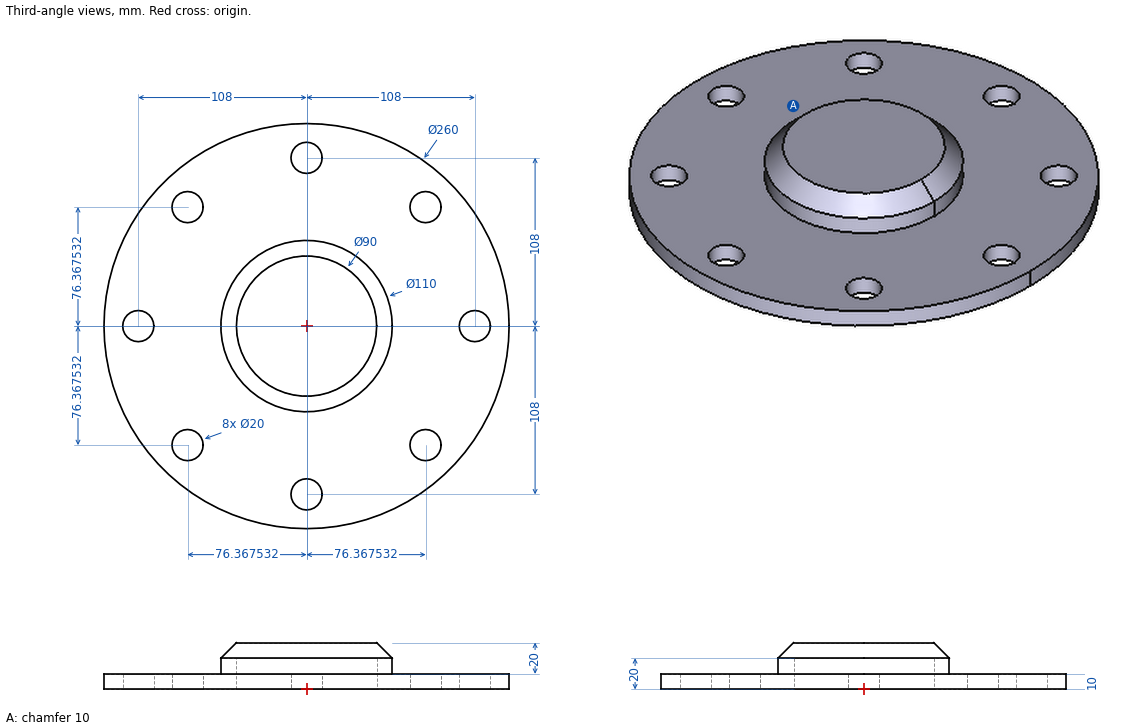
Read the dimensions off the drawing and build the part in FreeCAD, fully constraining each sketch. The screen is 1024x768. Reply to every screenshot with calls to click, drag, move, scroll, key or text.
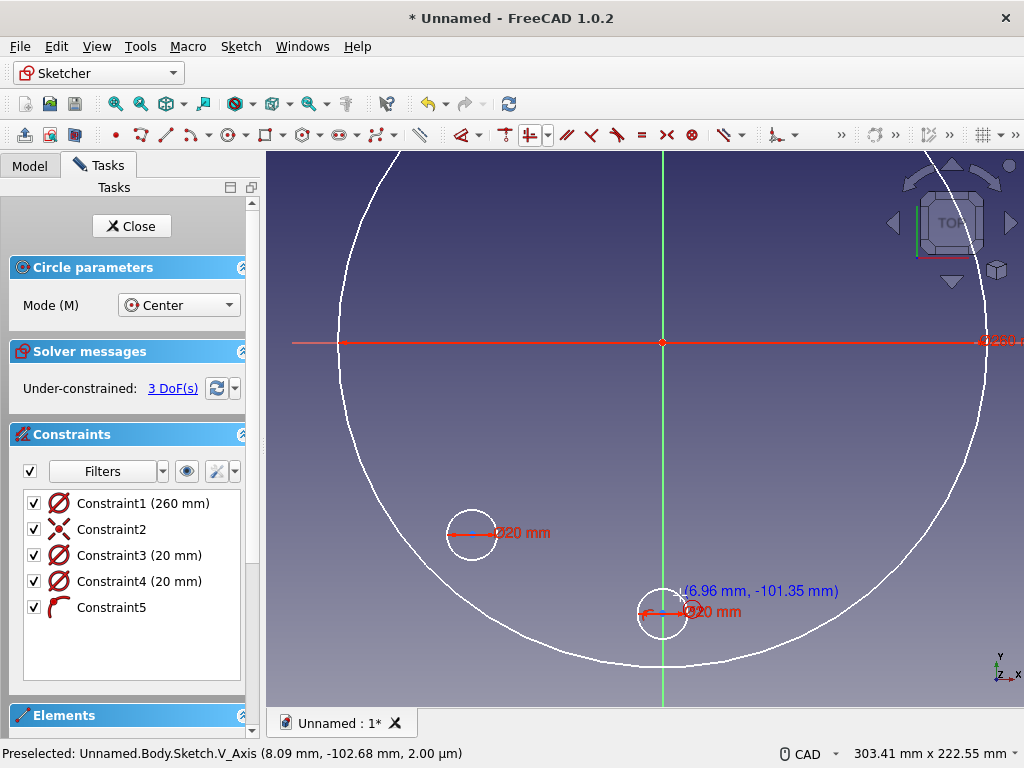
click(853, 534)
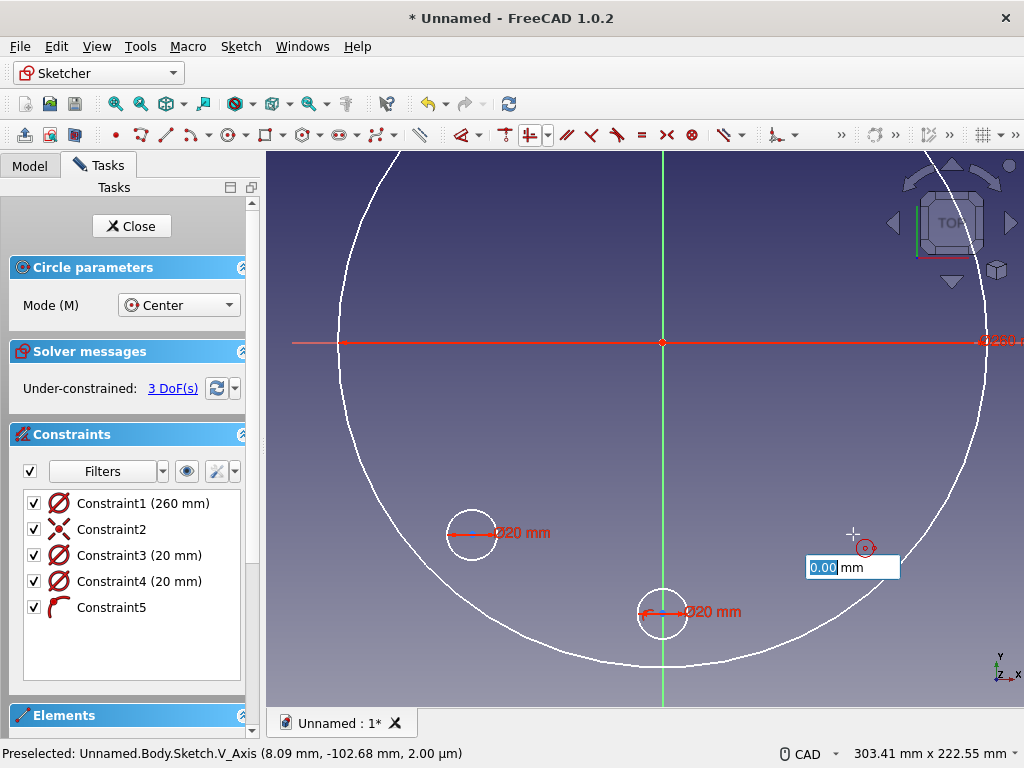
scroll(472, 534, down, 3)
move(691, 524)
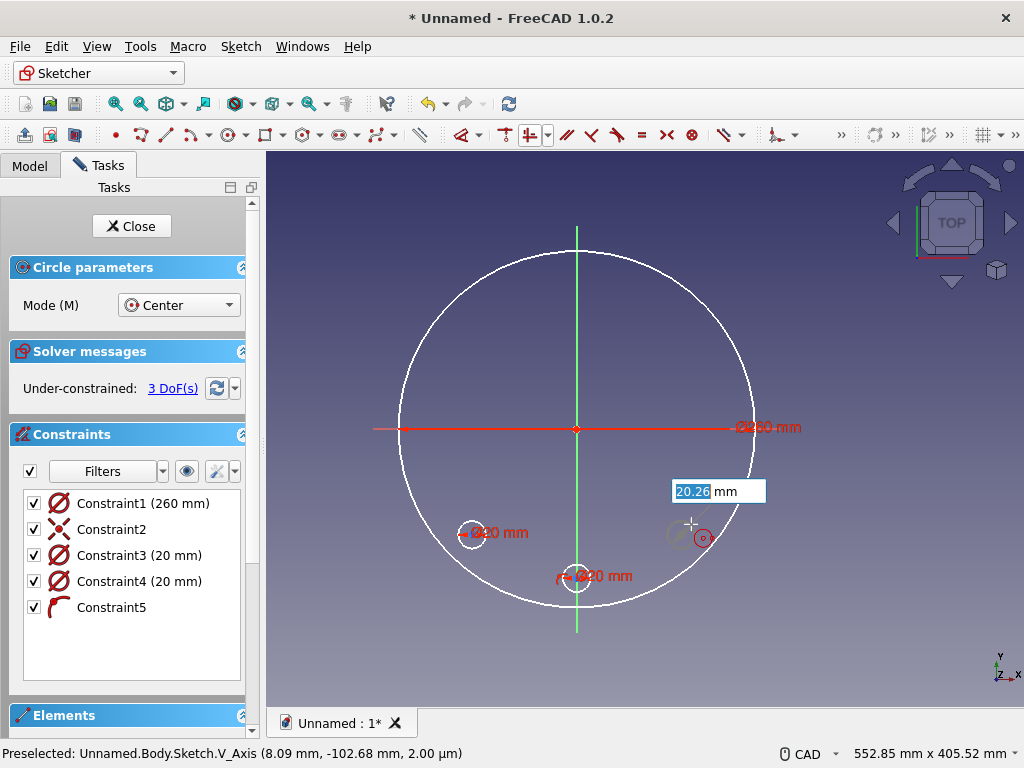
text(20)
key(Return)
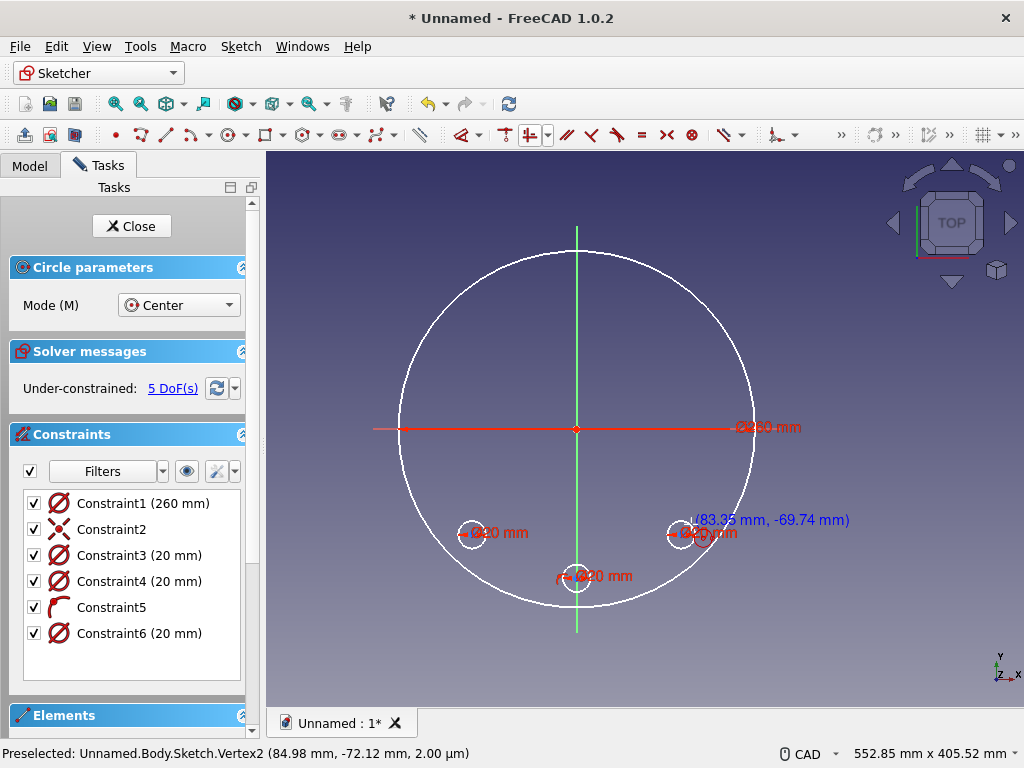
scroll(429, 429, up, 3)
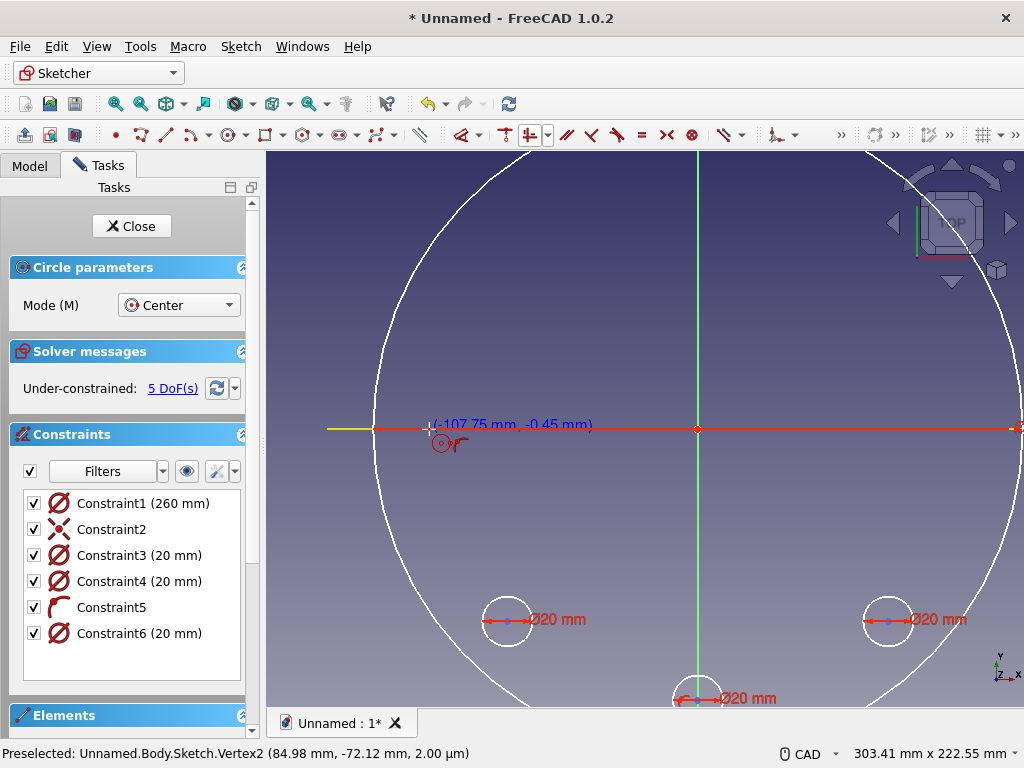
click(428, 429)
move(446, 412)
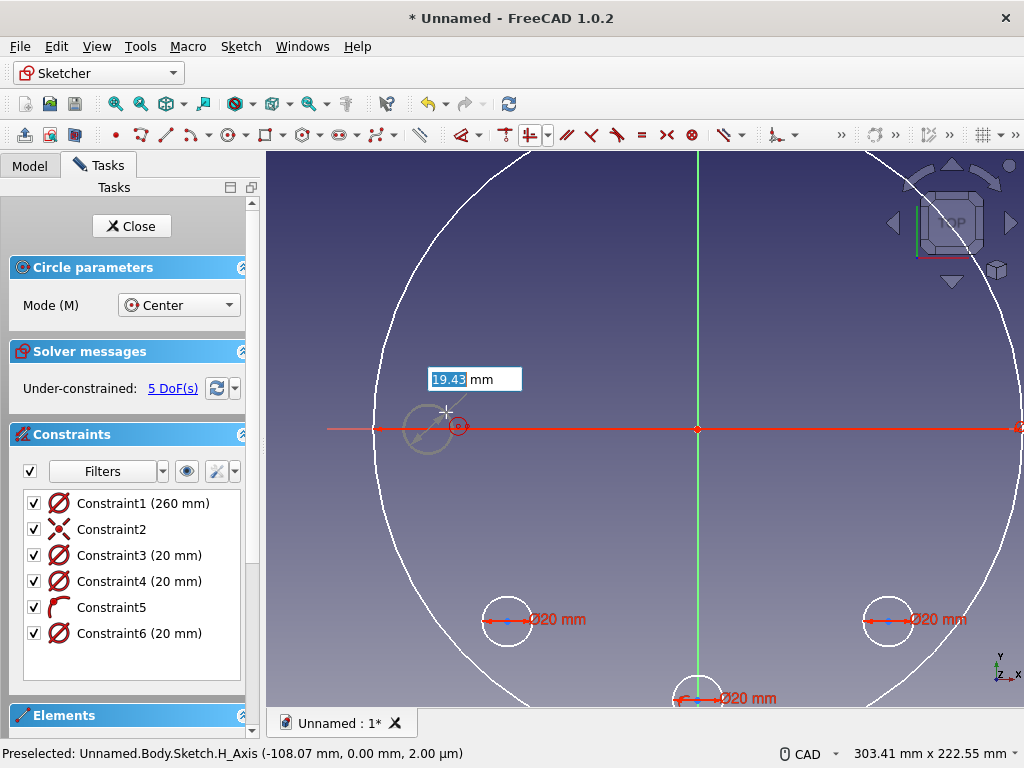
text(20)
key(Return)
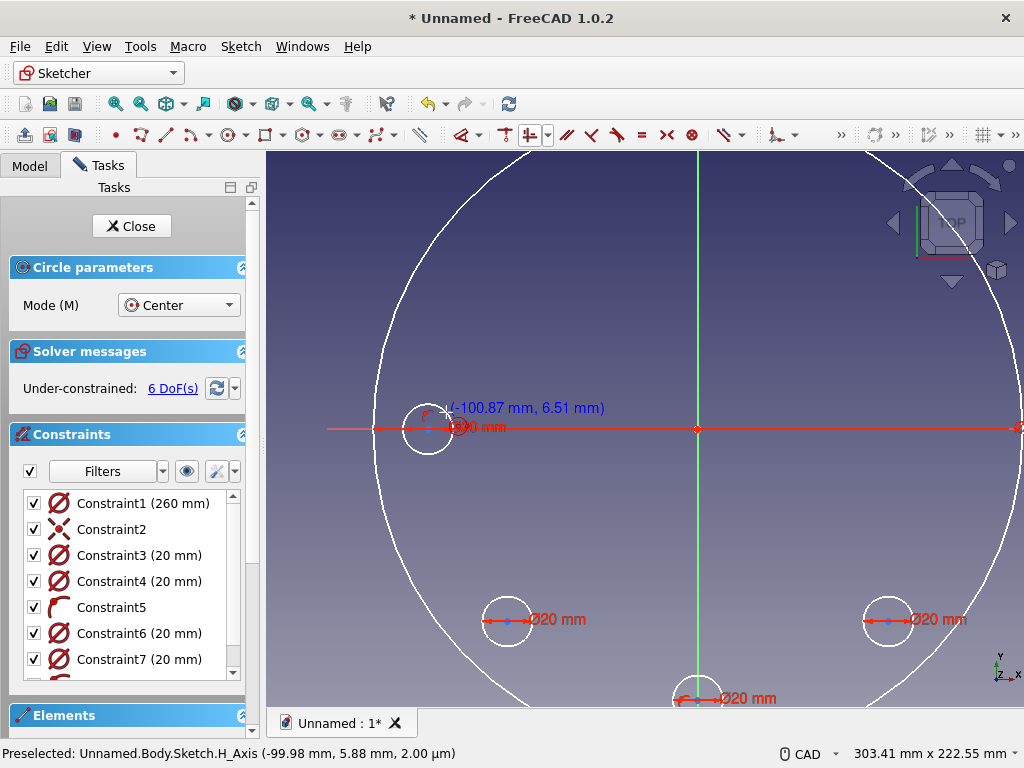
click(507, 238)
move(525, 221)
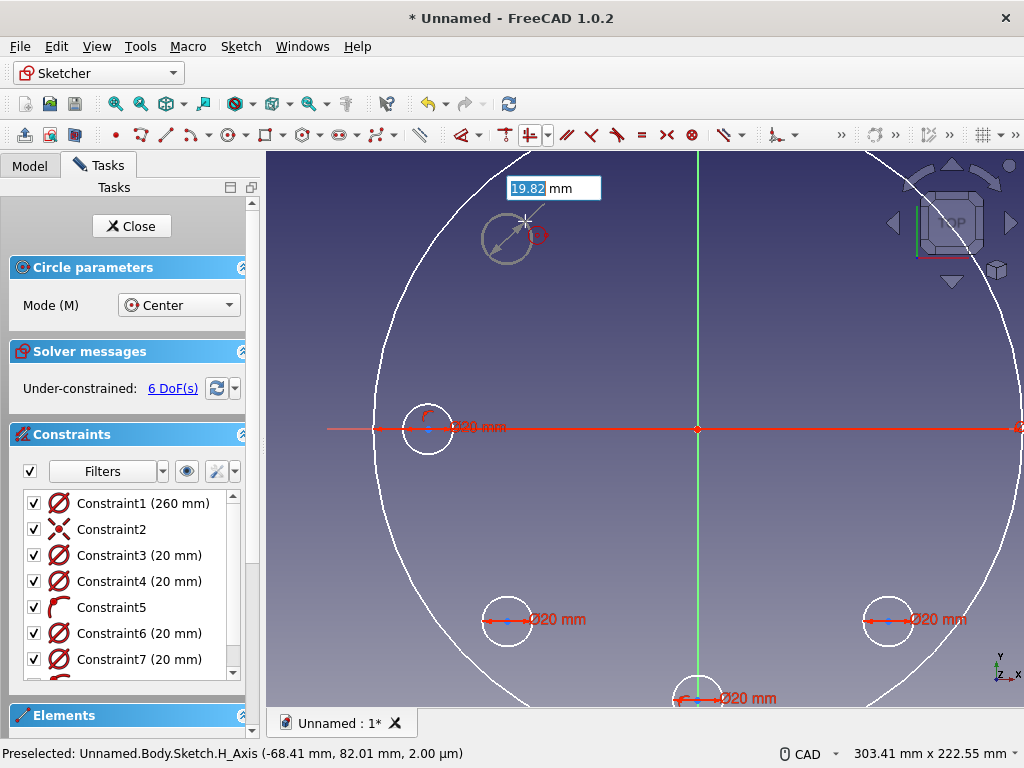
text(20)
key(Return)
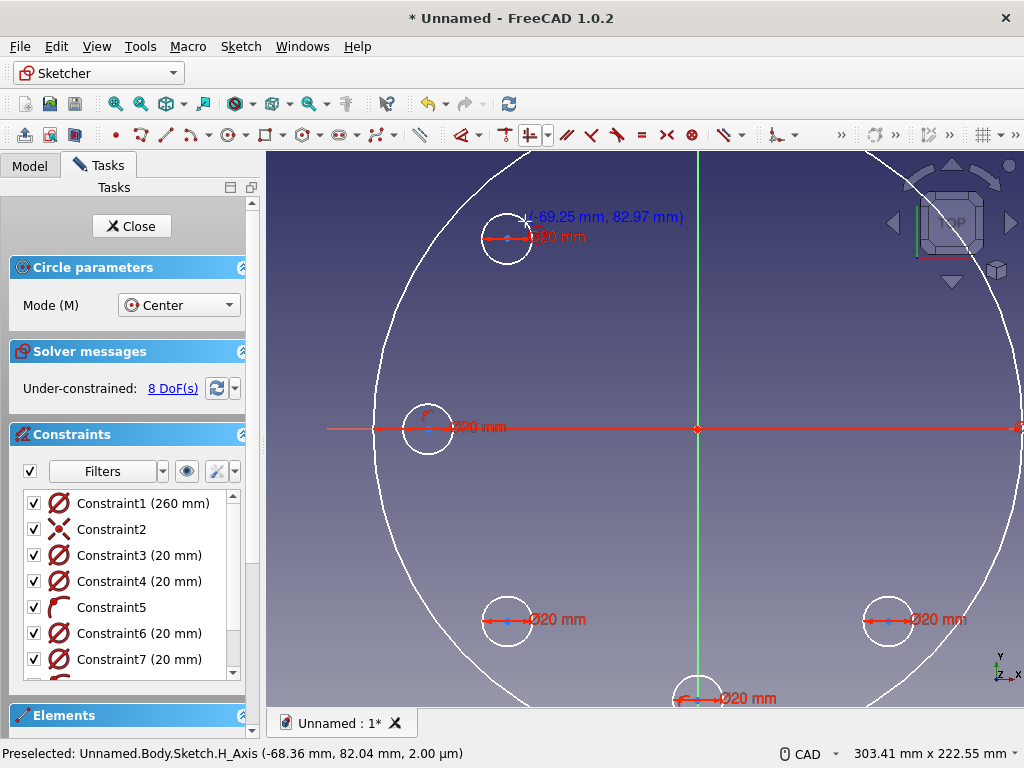
scroll(429, 429, down, 3)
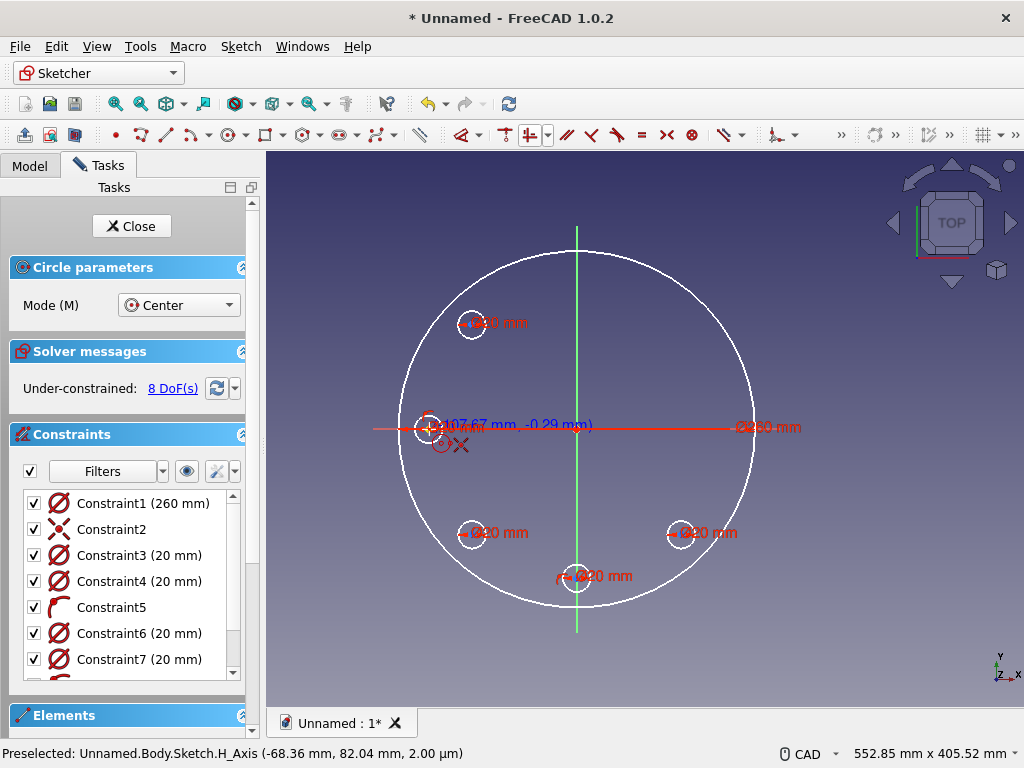
scroll(725, 429, up, 3)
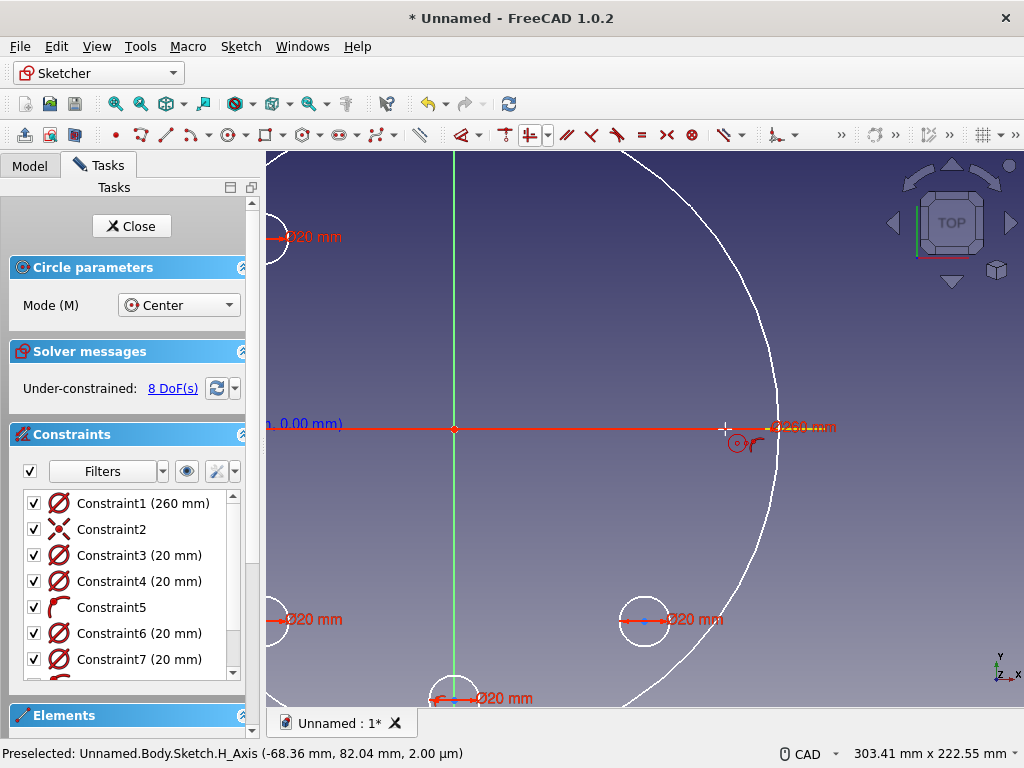
click(724, 429)
move(742, 412)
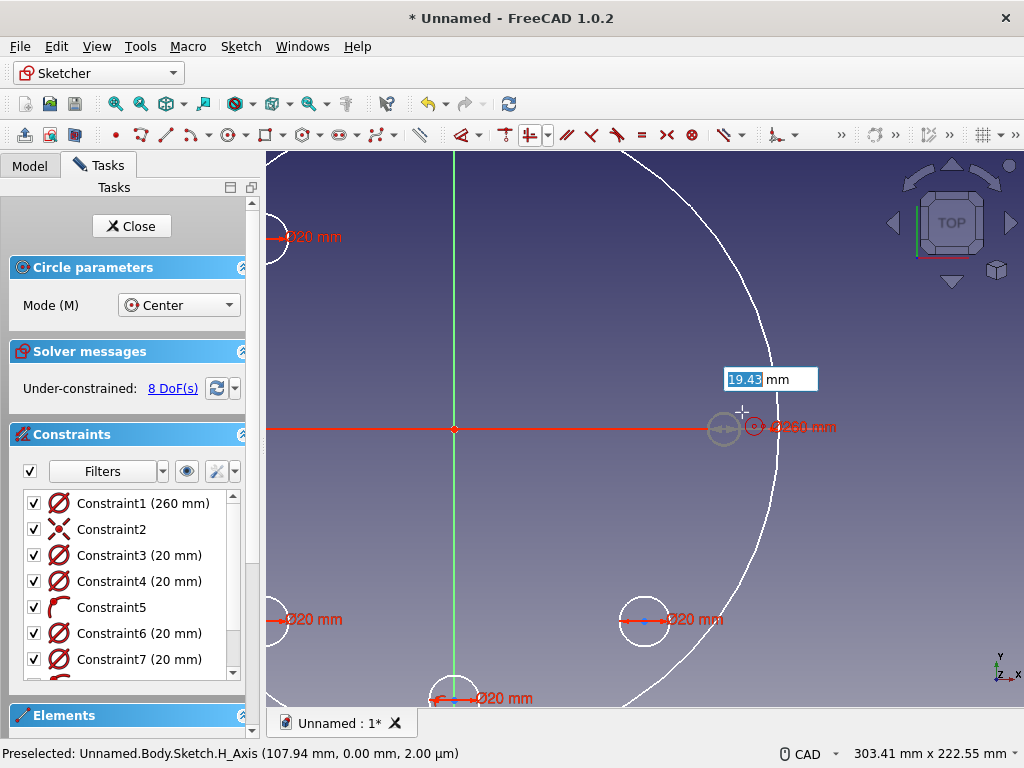
text(20)
key(Return)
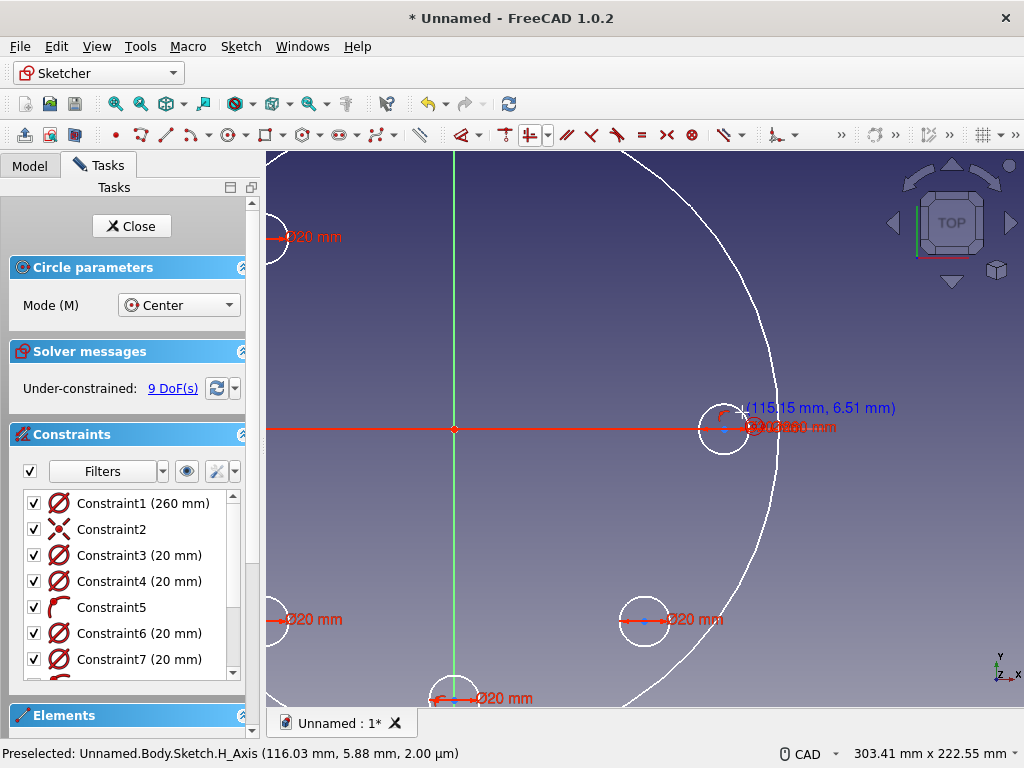
scroll(725, 429, down, 3)